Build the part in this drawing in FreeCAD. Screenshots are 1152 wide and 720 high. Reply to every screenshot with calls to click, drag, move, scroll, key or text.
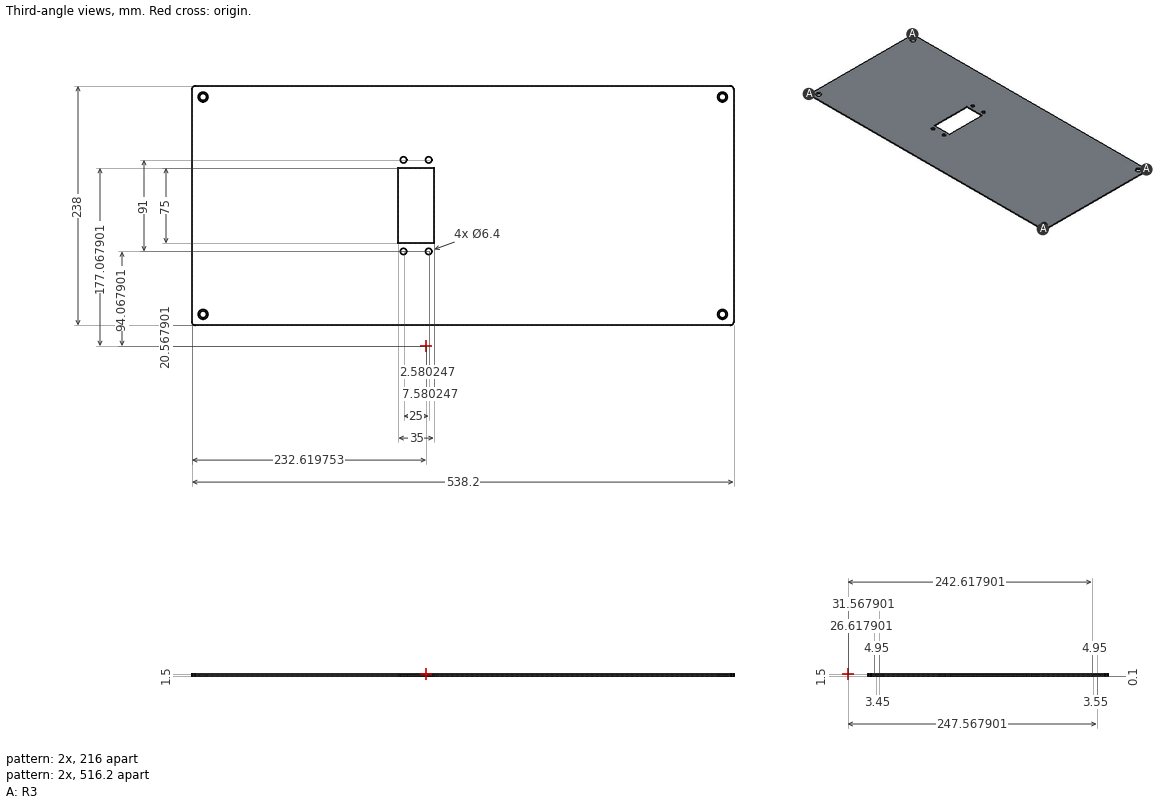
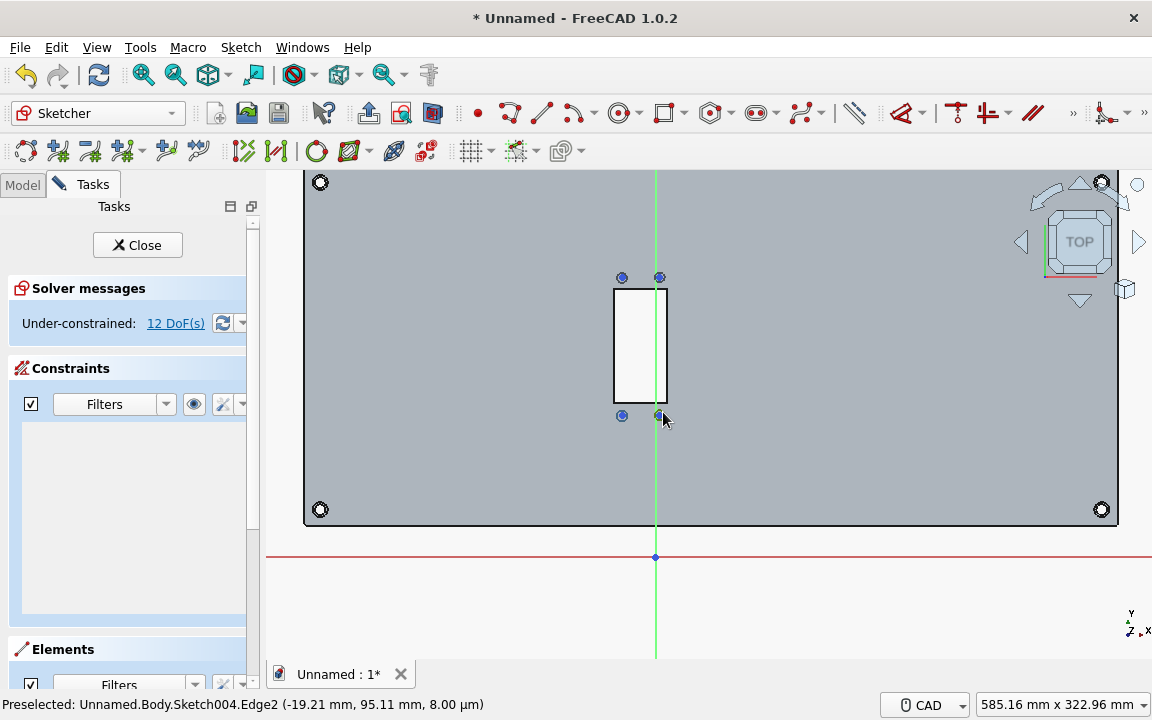
scroll(663, 274, up, 6)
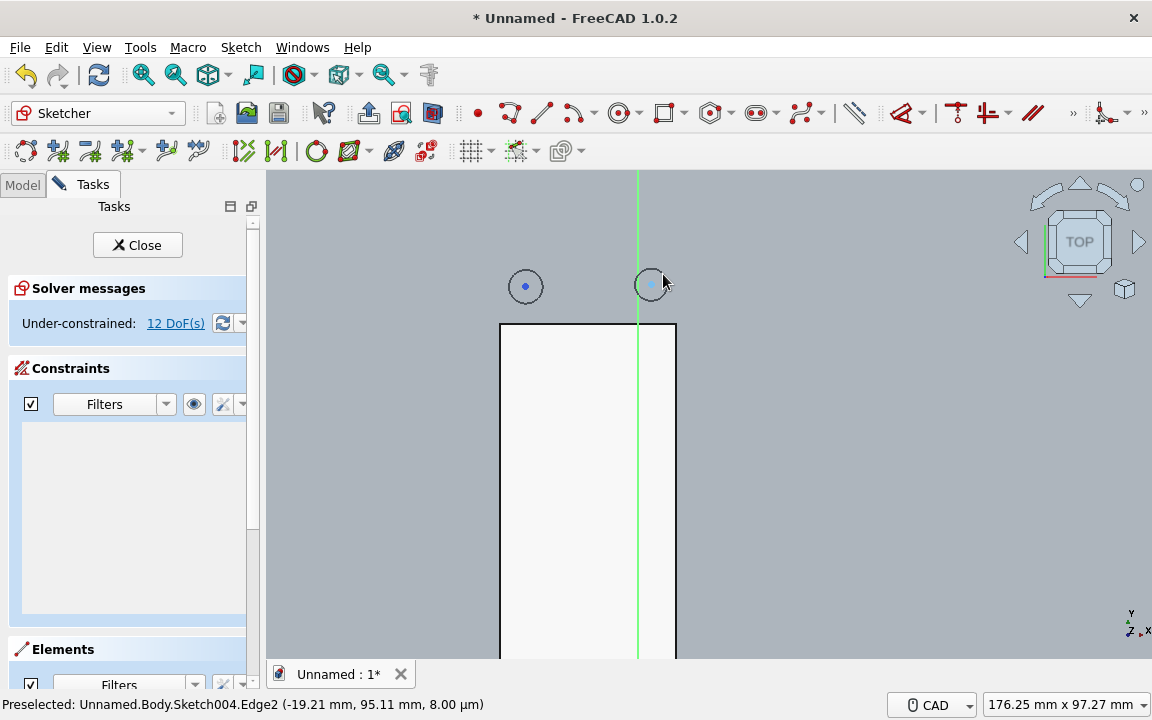
click(663, 273)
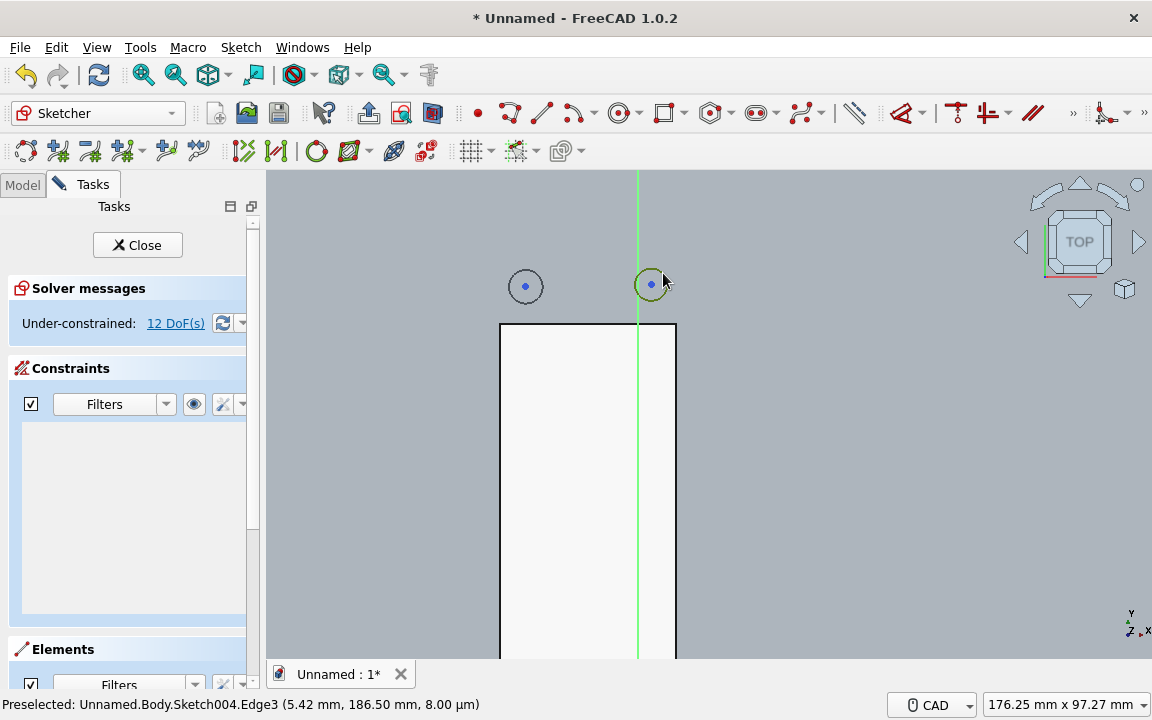
click(538, 275)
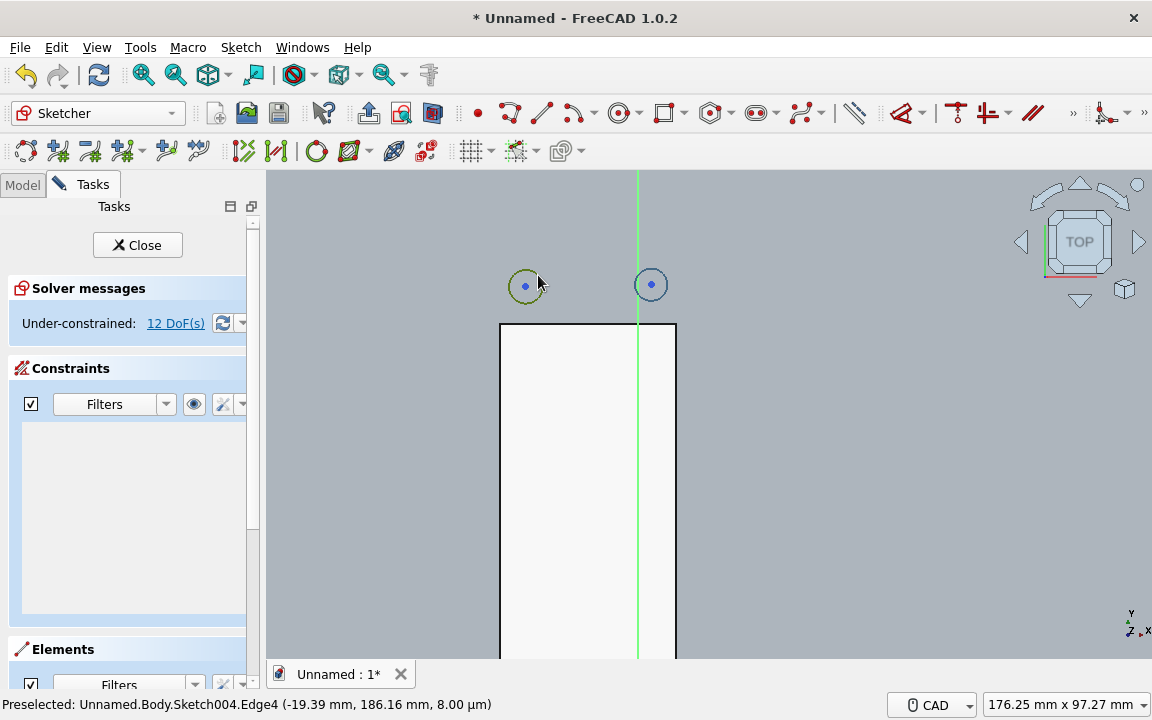
key(e)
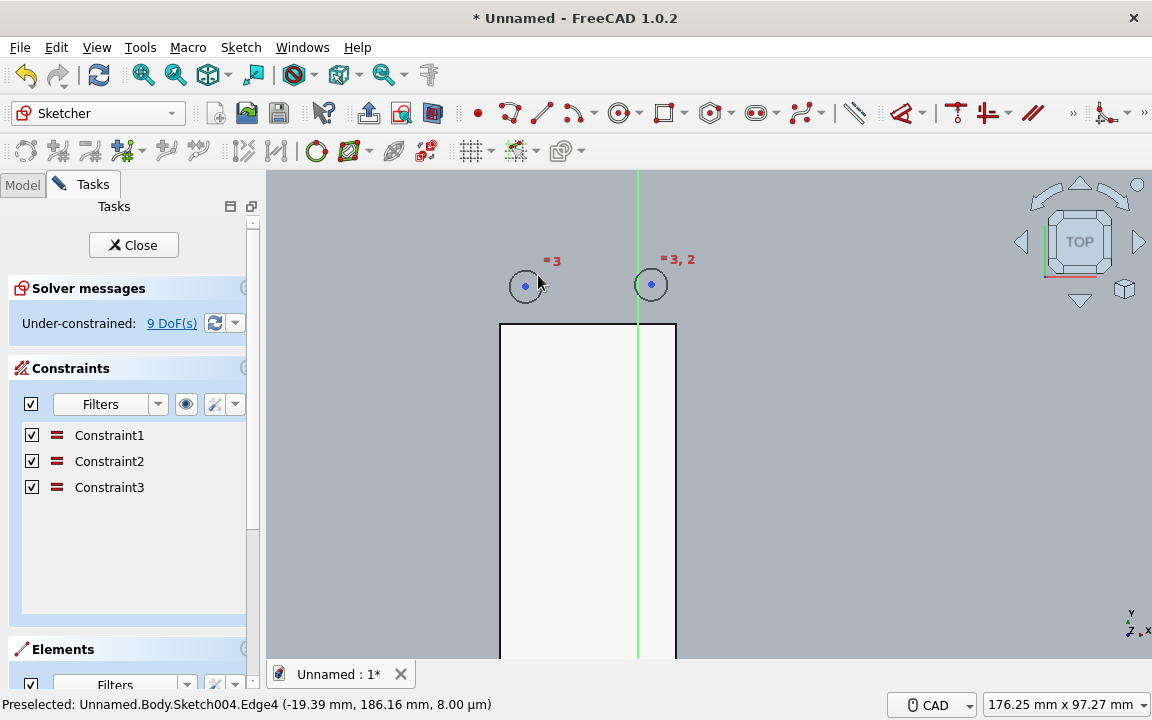
scroll(663, 274, down, 6)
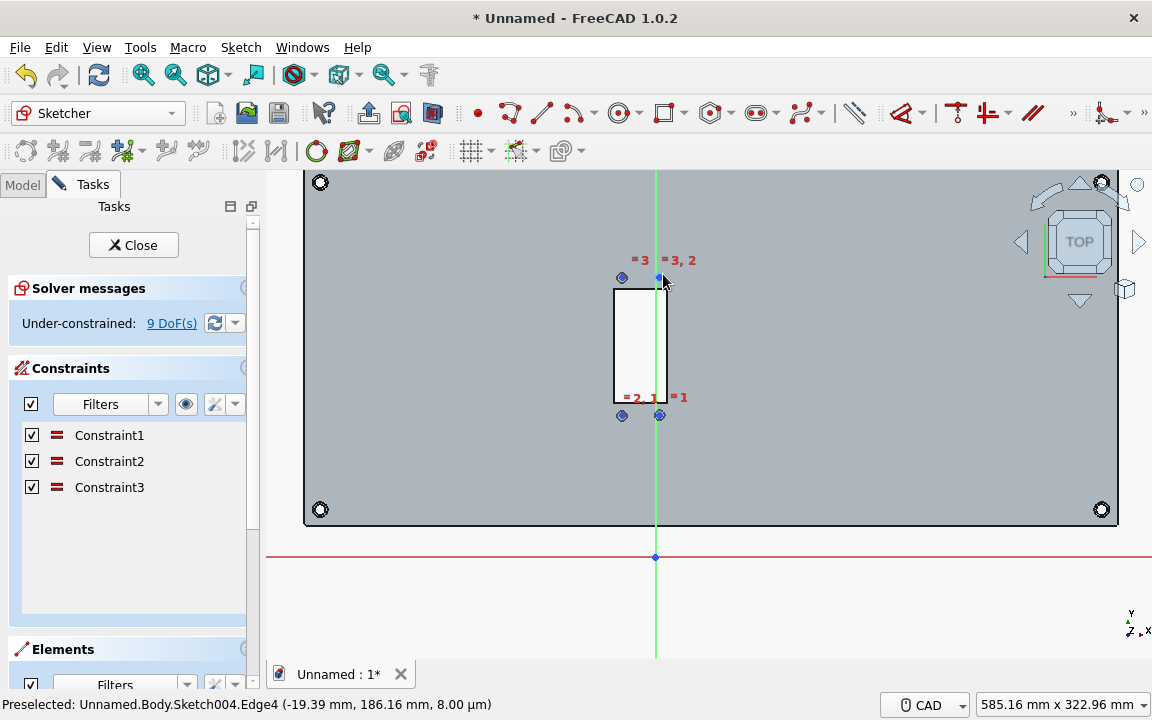
click(660, 415)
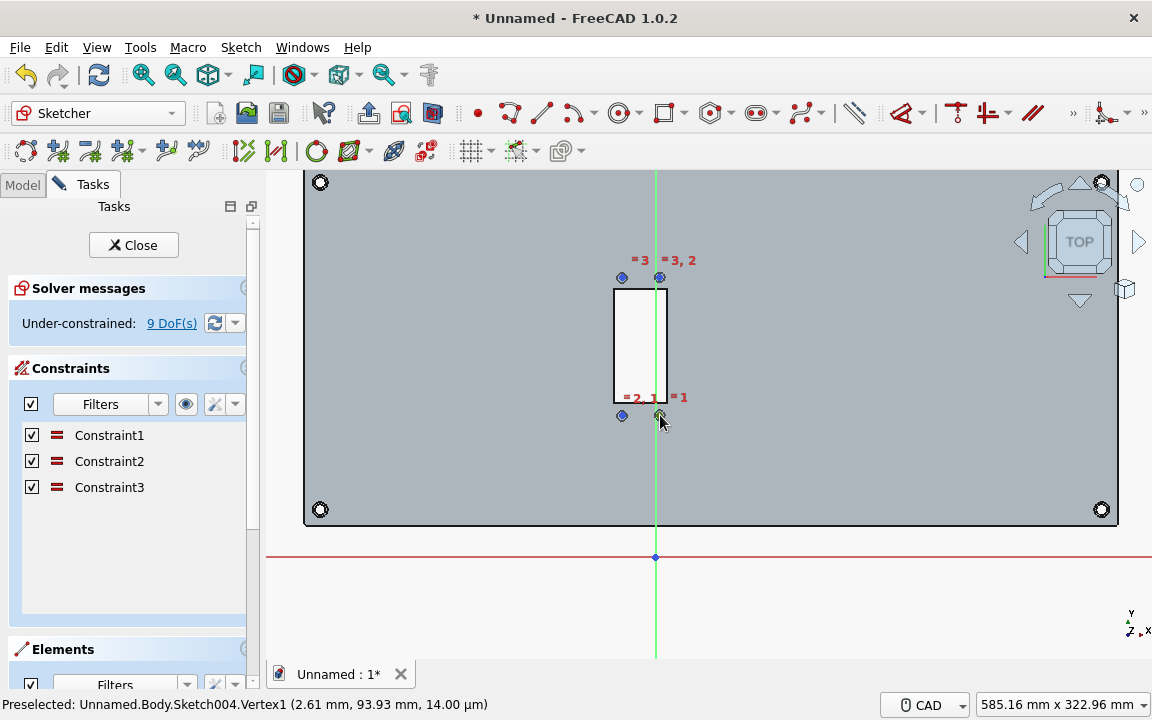
click(622, 416)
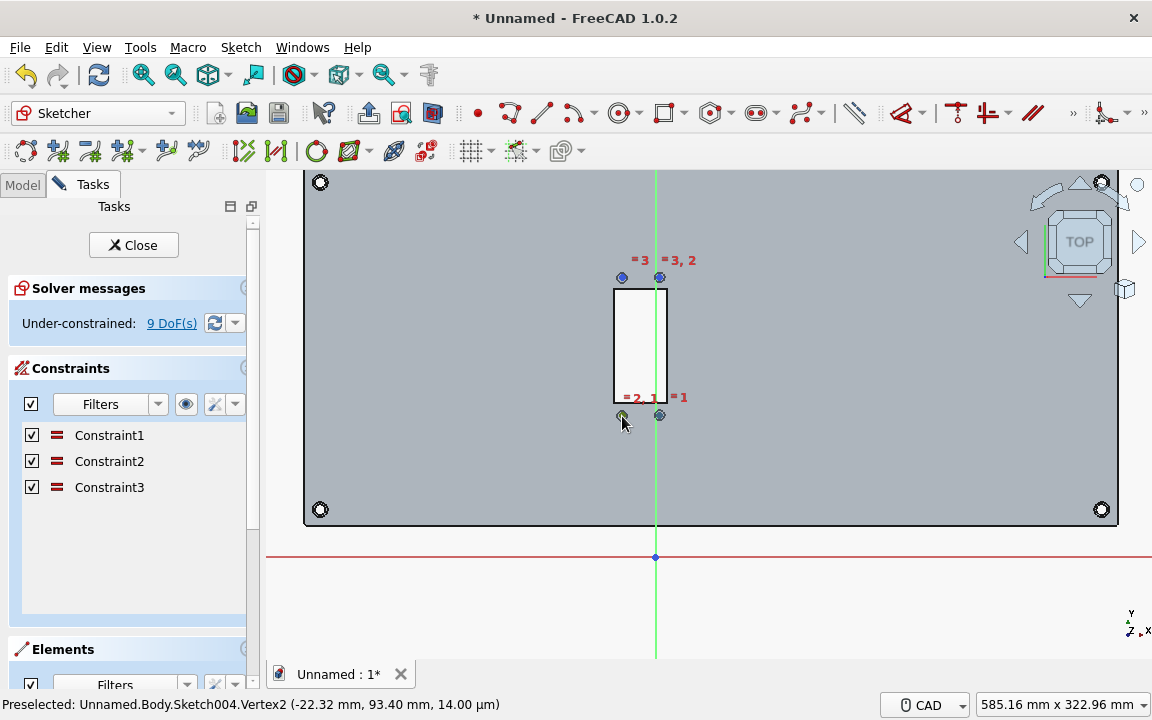
click(1010, 114)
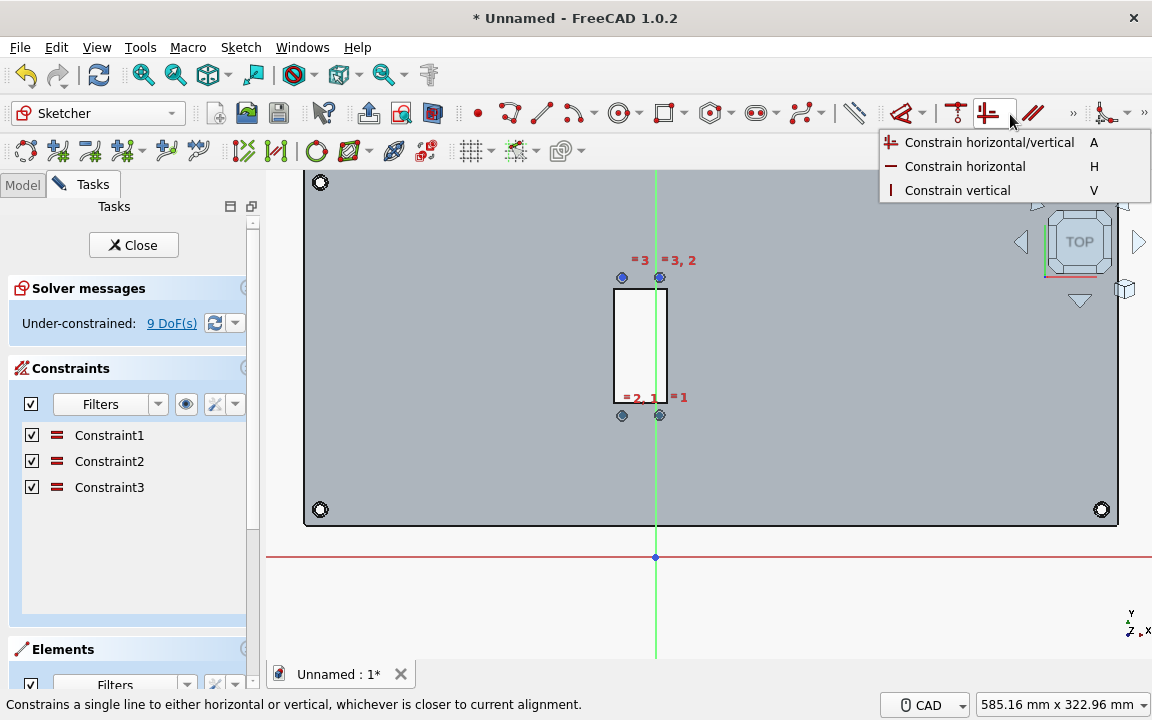
click(1015, 166)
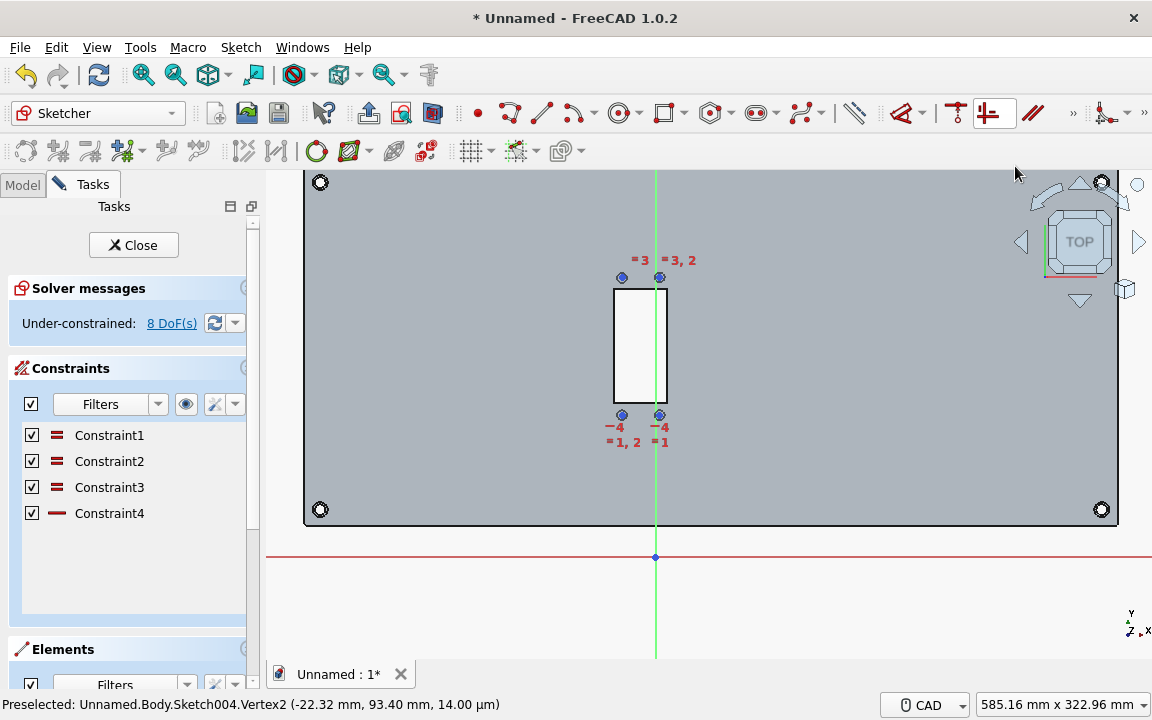
click(660, 415)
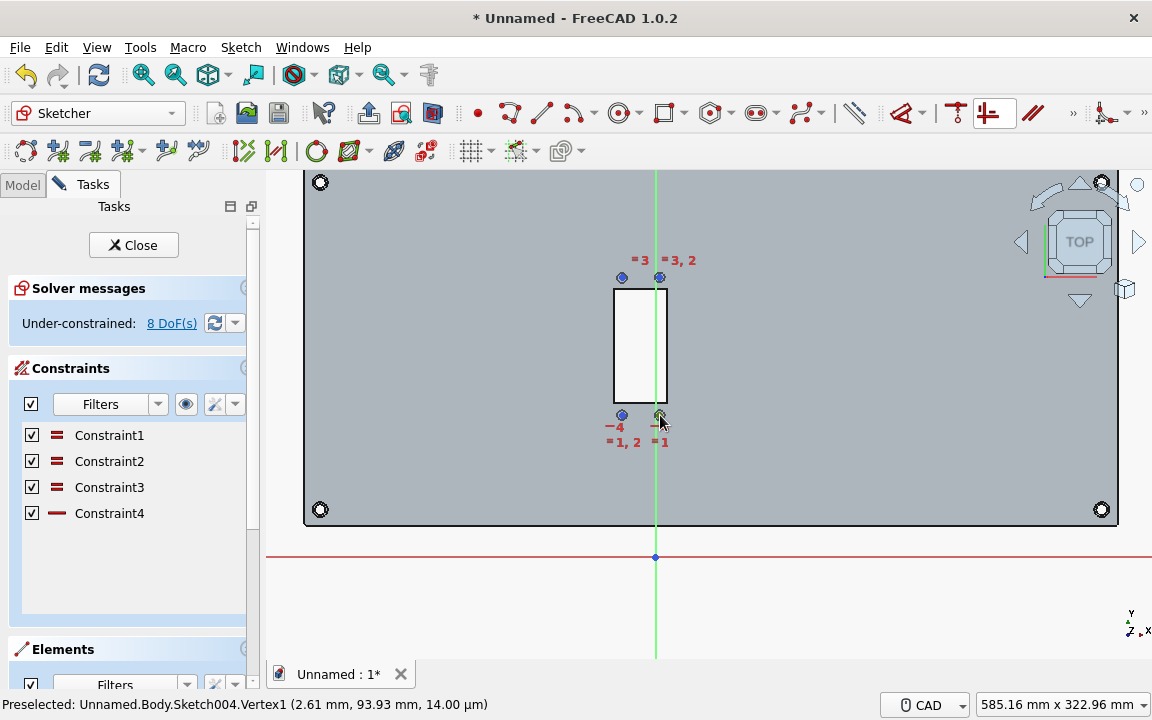
click(660, 277)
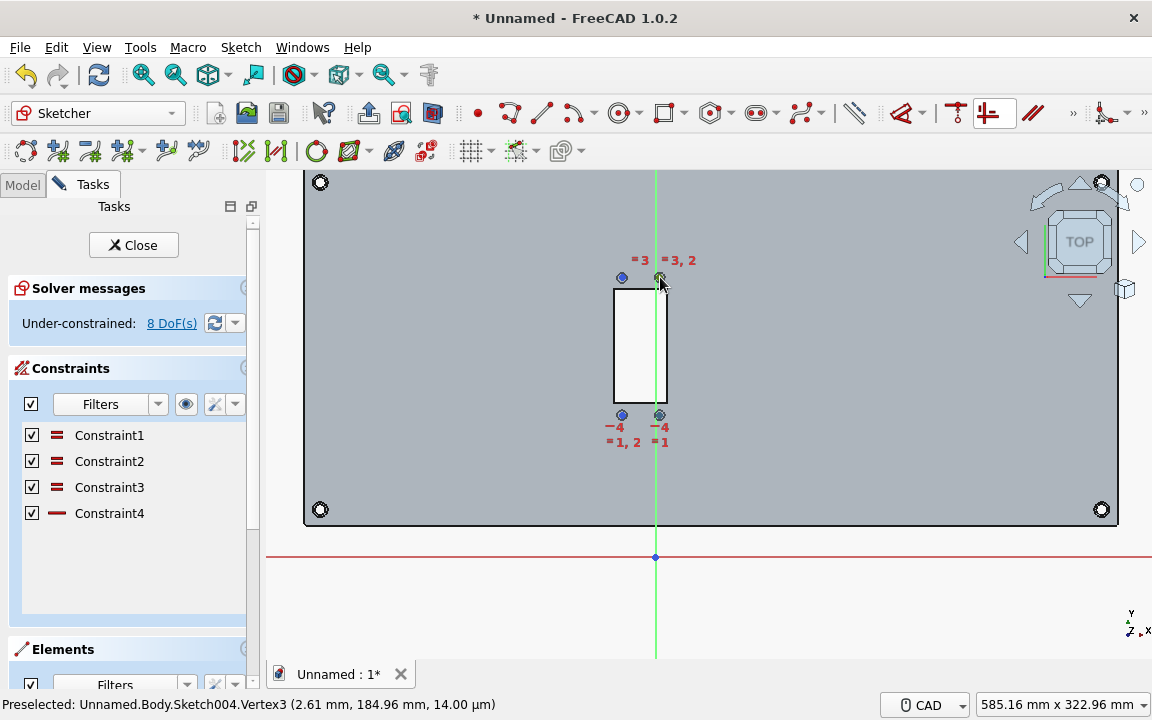
key(v)